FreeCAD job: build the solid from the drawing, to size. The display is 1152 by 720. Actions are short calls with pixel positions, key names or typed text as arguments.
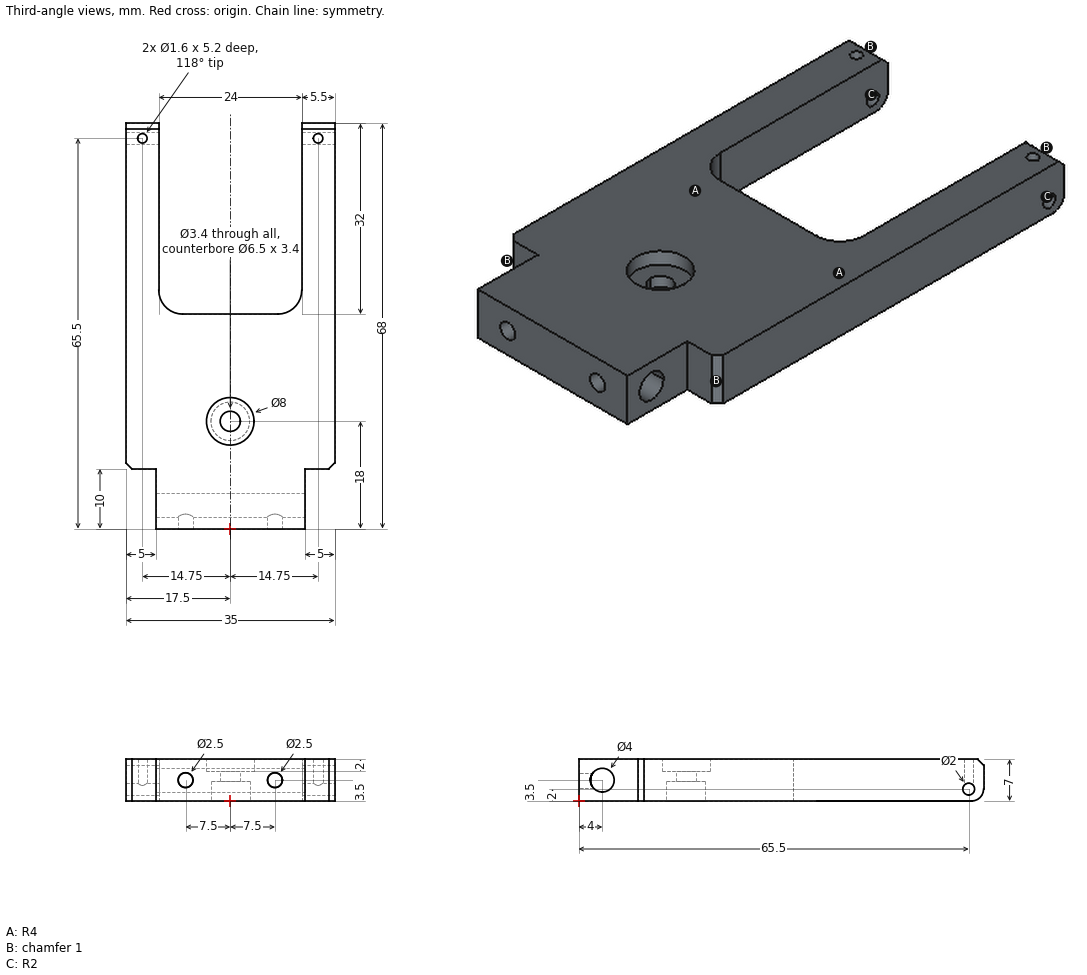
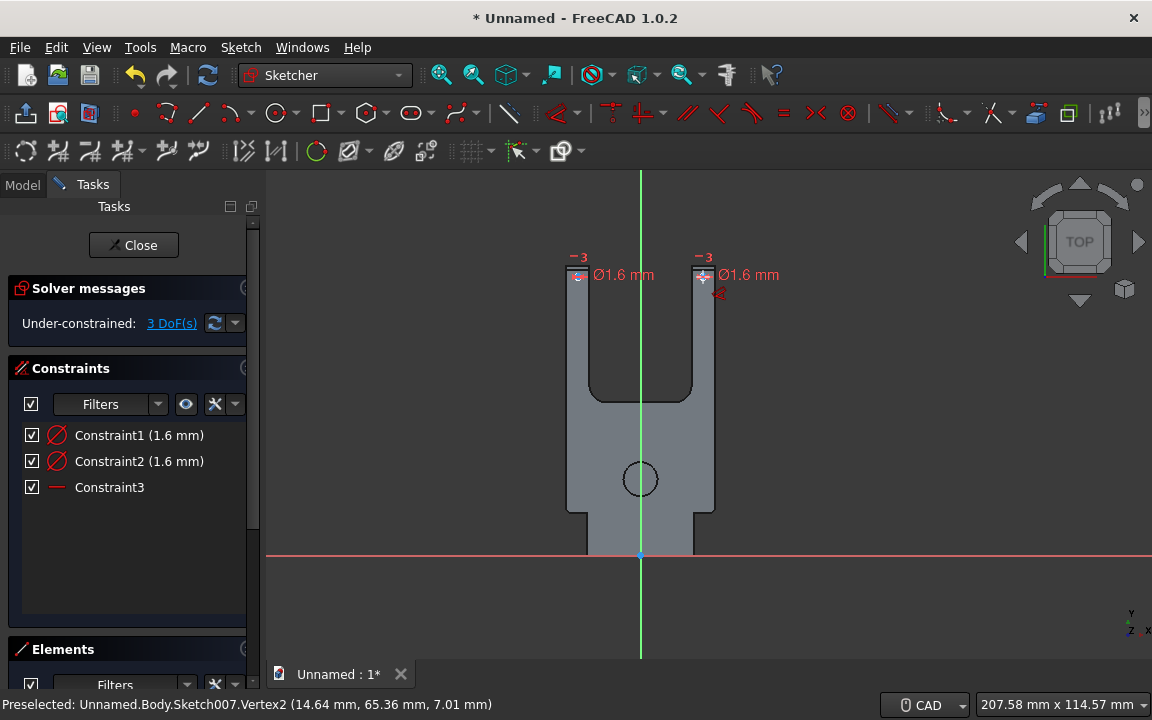
click(578, 277)
click(544, 416)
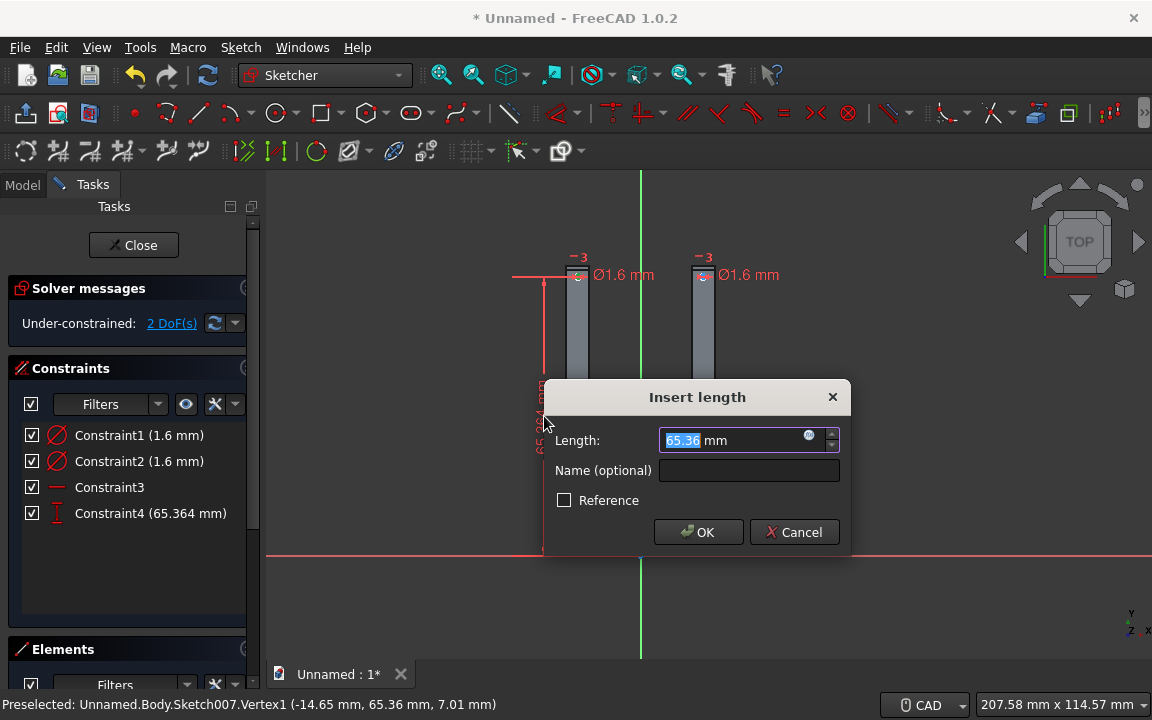
text(65.5)
key(Return)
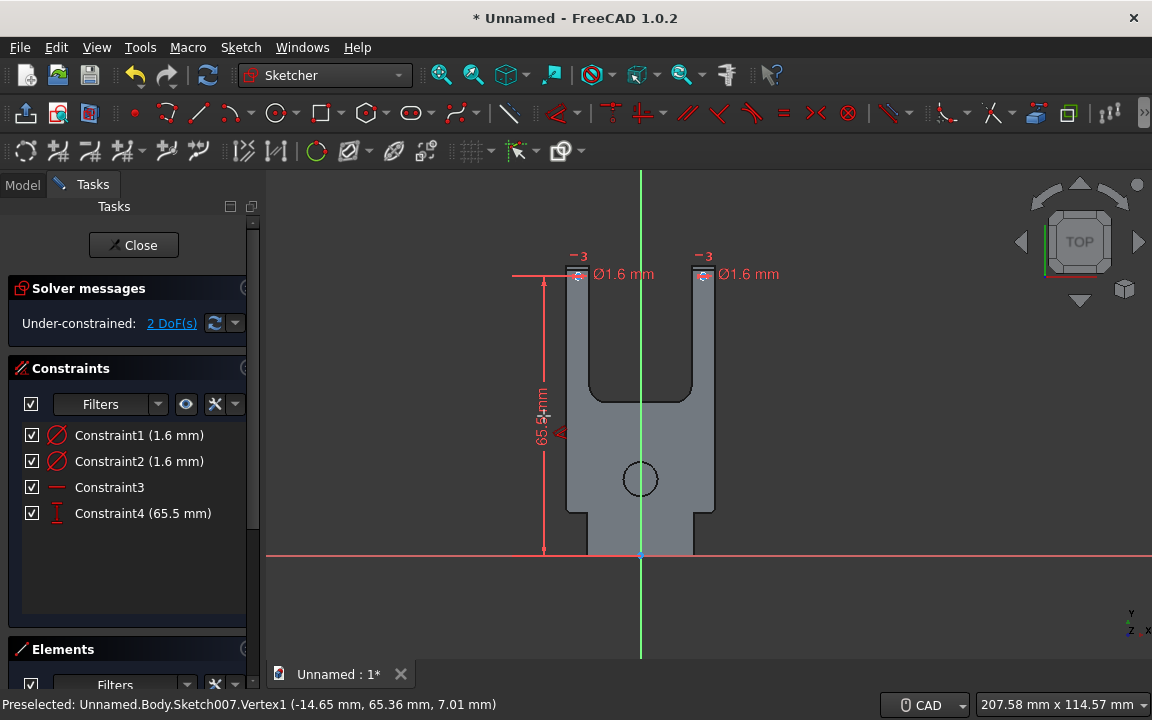
click(578, 276)
click(609, 590)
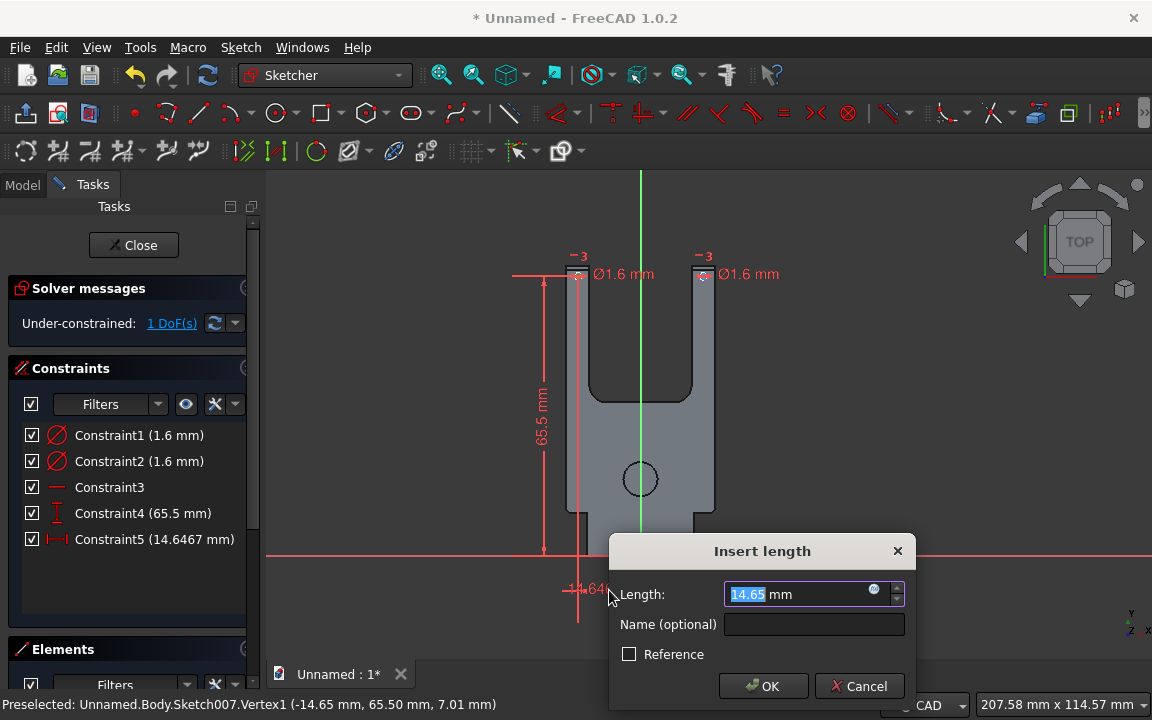
text(14.75)
key(Return)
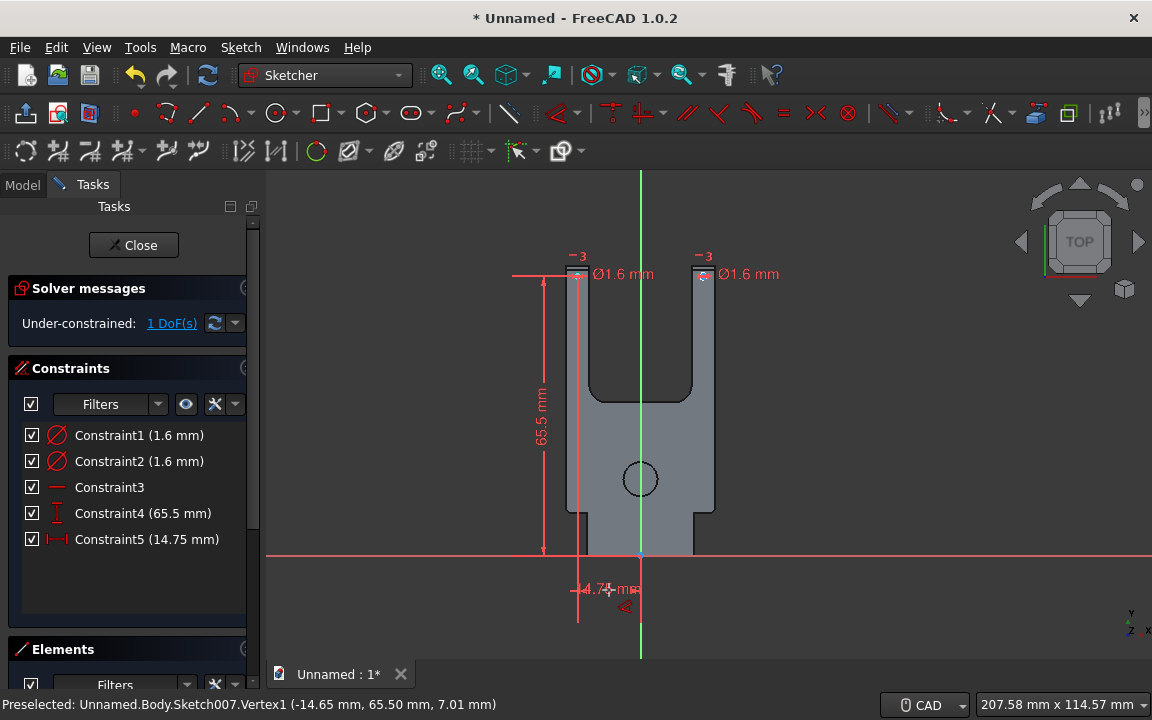
click(703, 276)
click(686, 590)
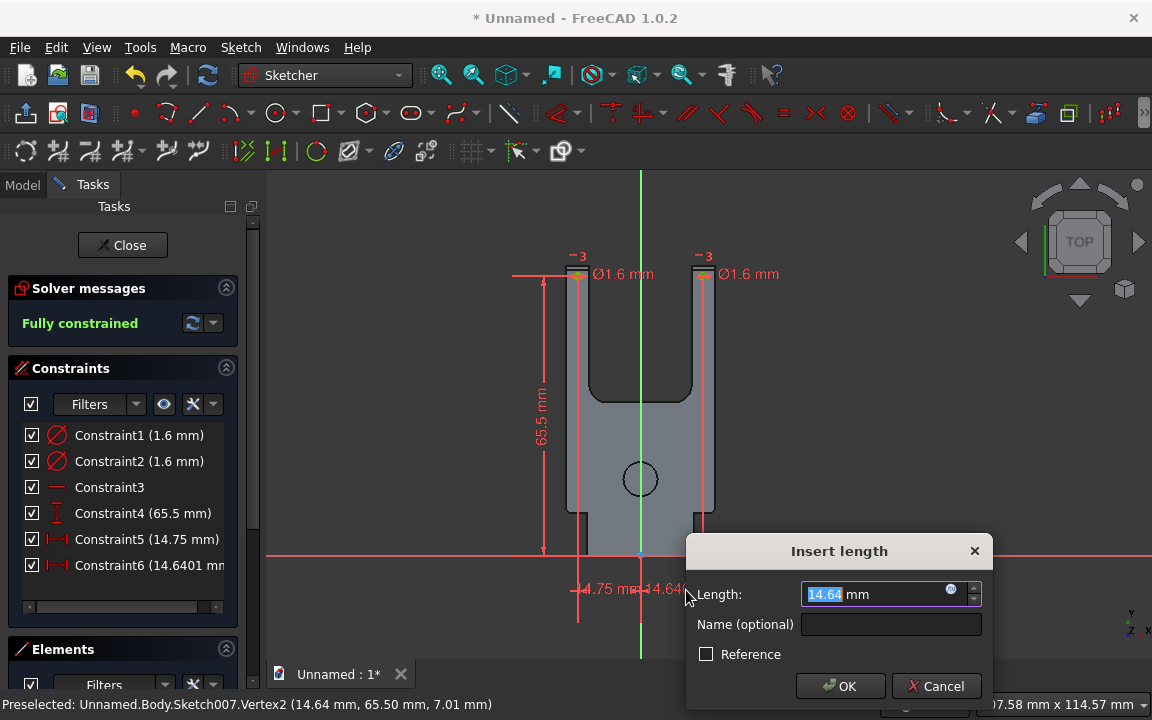
text(14.75)
key(Return)
key(Escape)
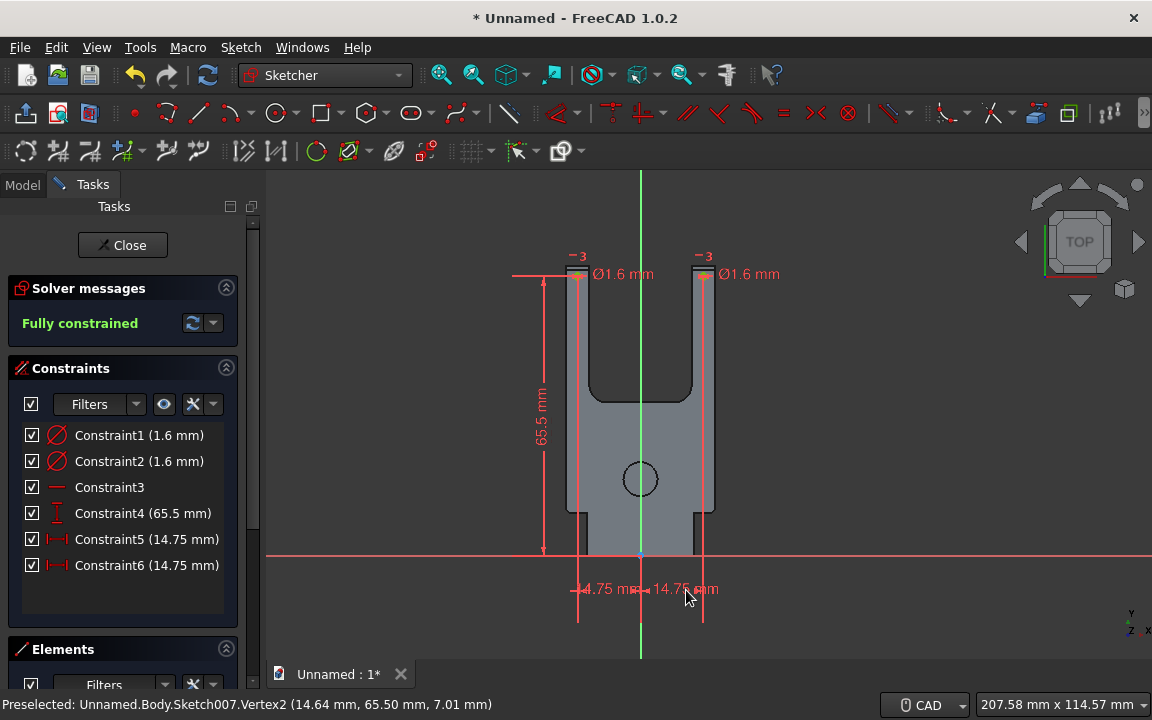
click(123, 245)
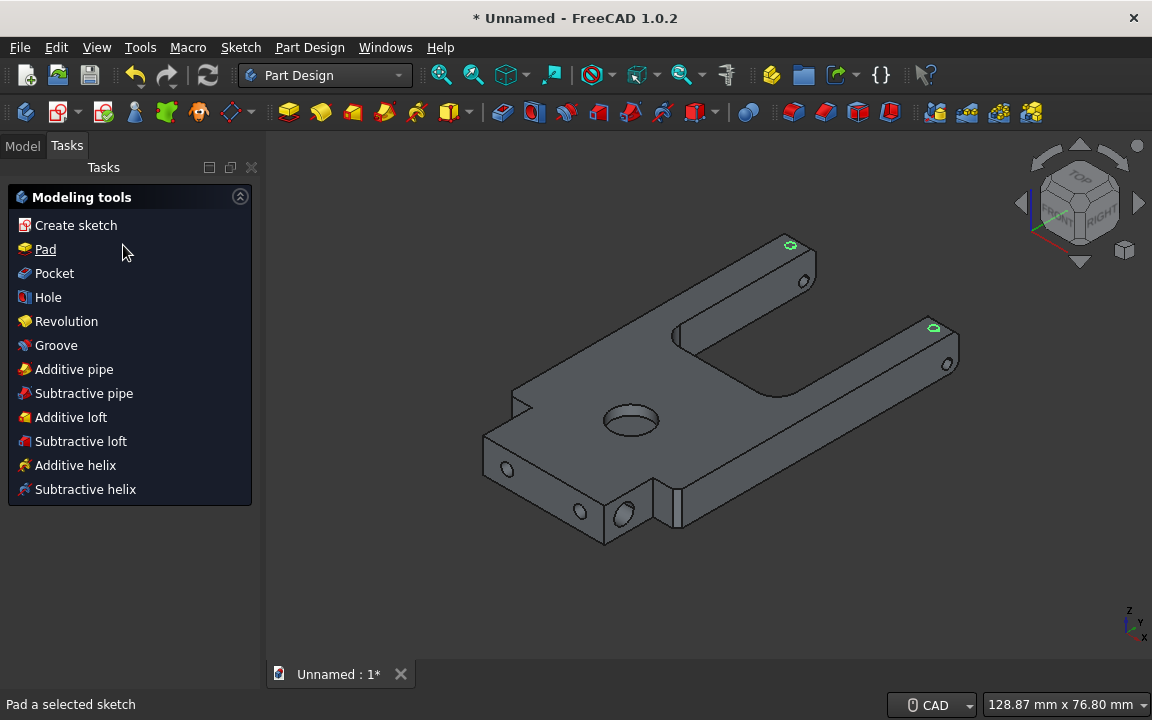
click(536, 112)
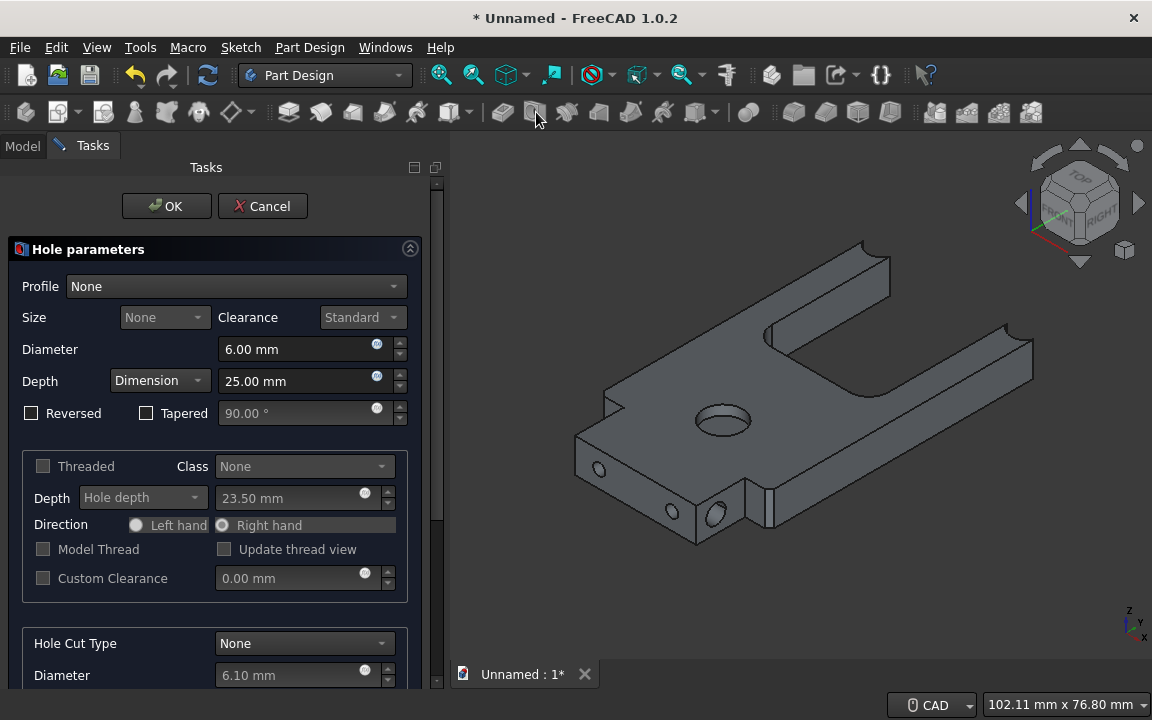
triple_click(305, 349)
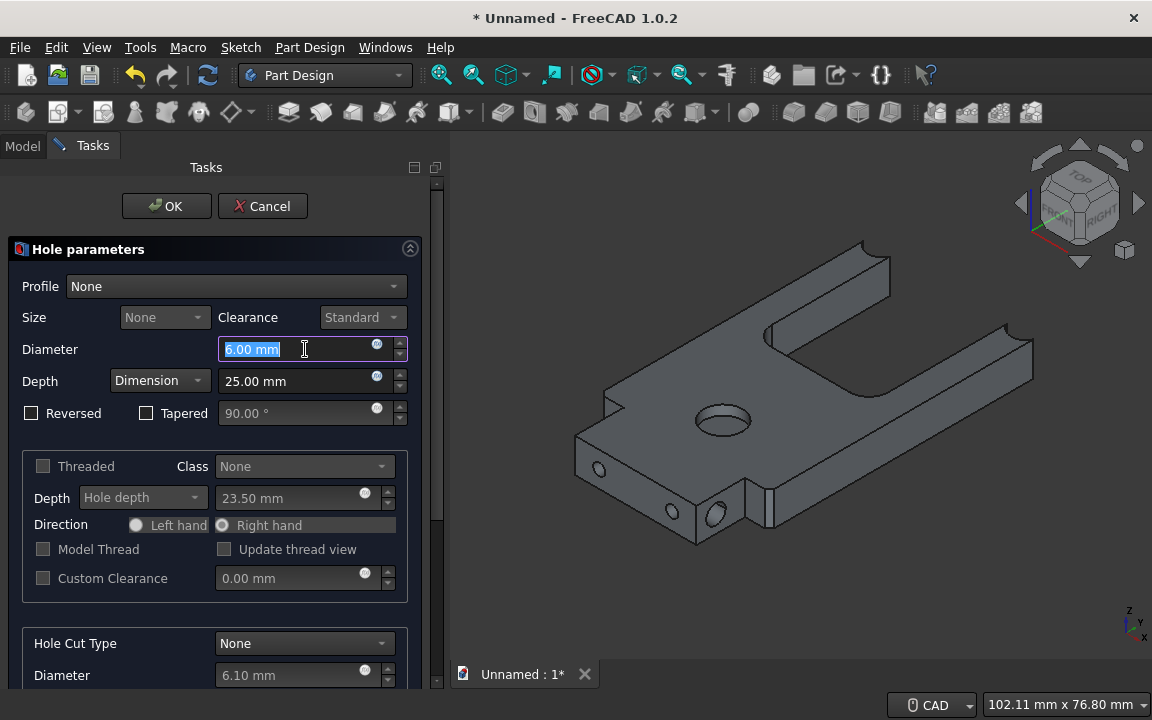
text(1.6)
key(Tab)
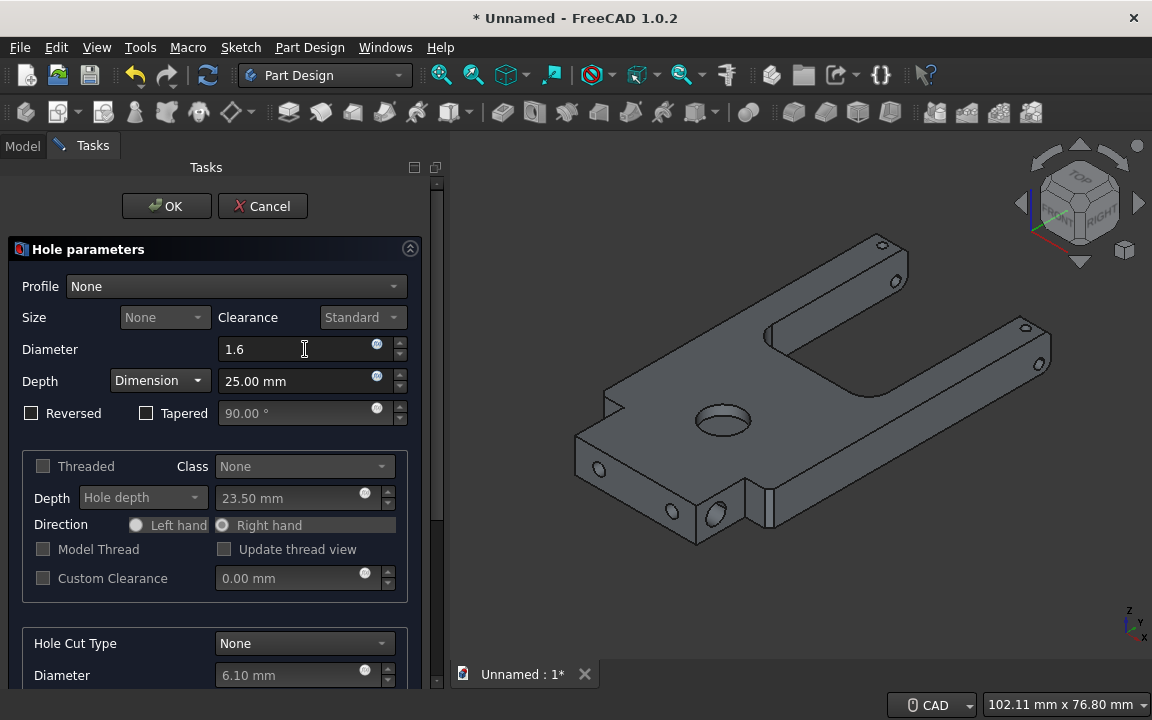
triple_click(305, 381)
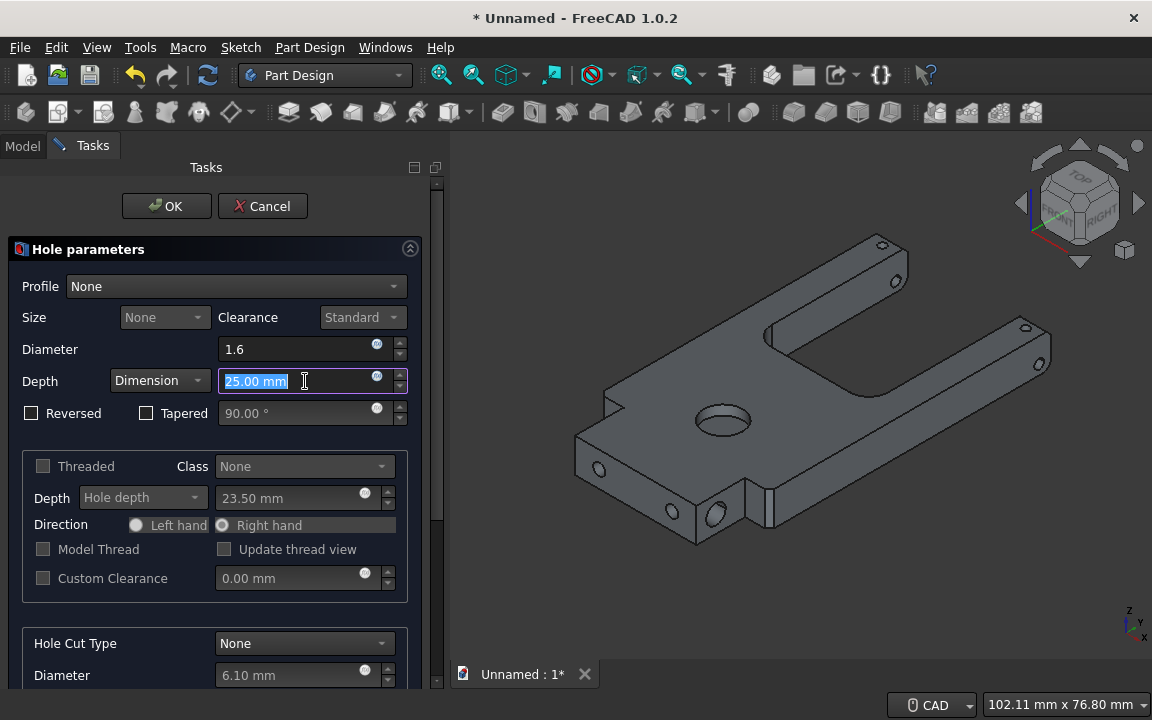
text(5.2)
key(Tab)